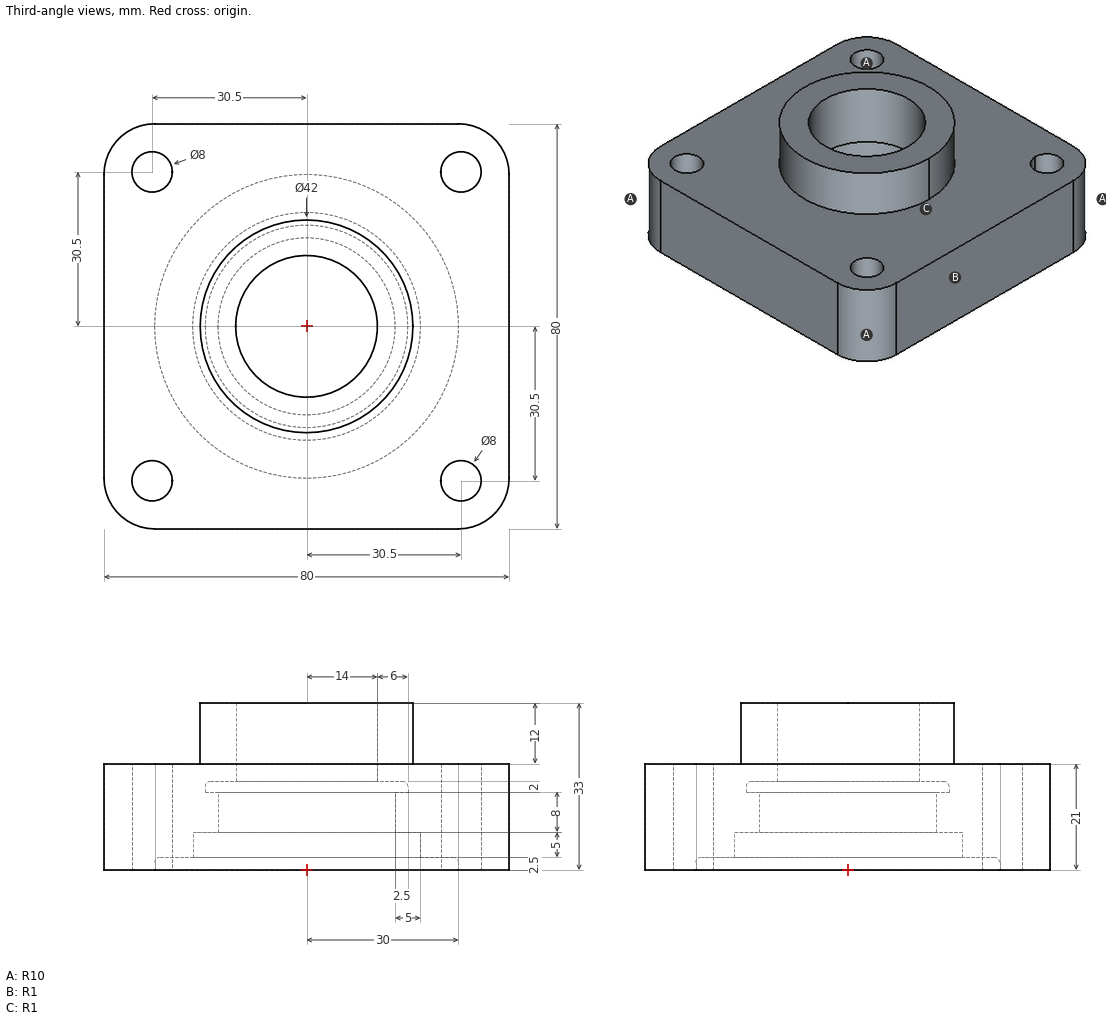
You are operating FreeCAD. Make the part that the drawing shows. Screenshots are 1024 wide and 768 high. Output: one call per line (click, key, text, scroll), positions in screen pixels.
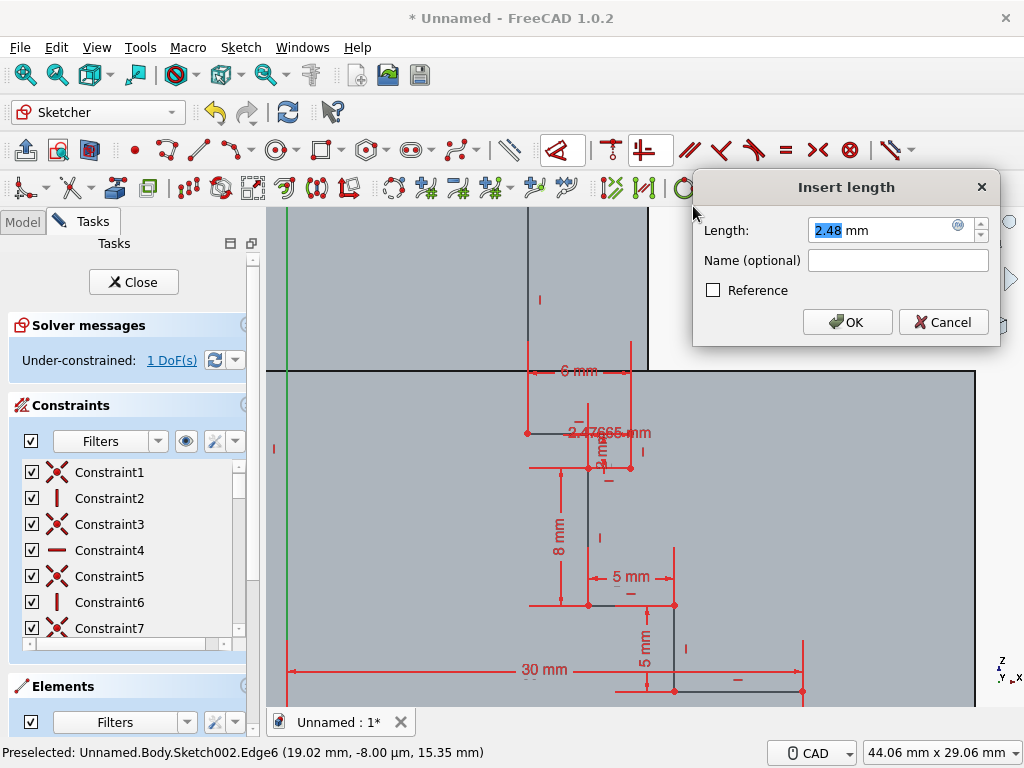
text(2.5)
key(Return)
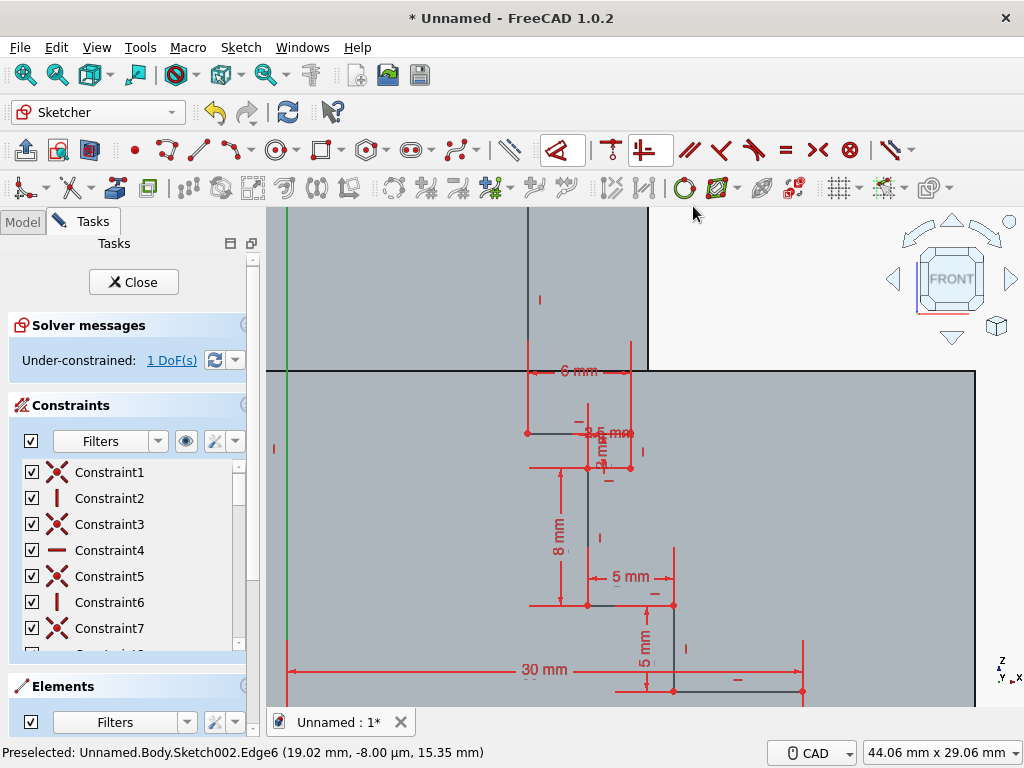
scroll(615, 467, down, 3)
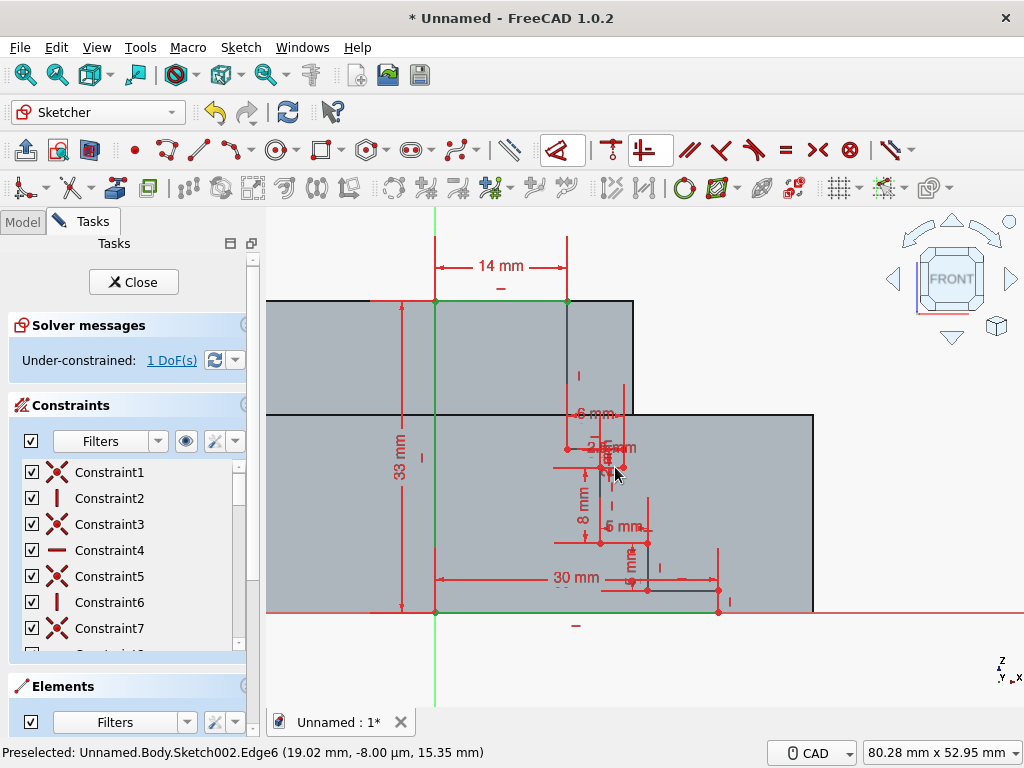
scroll(718, 597, up, 4)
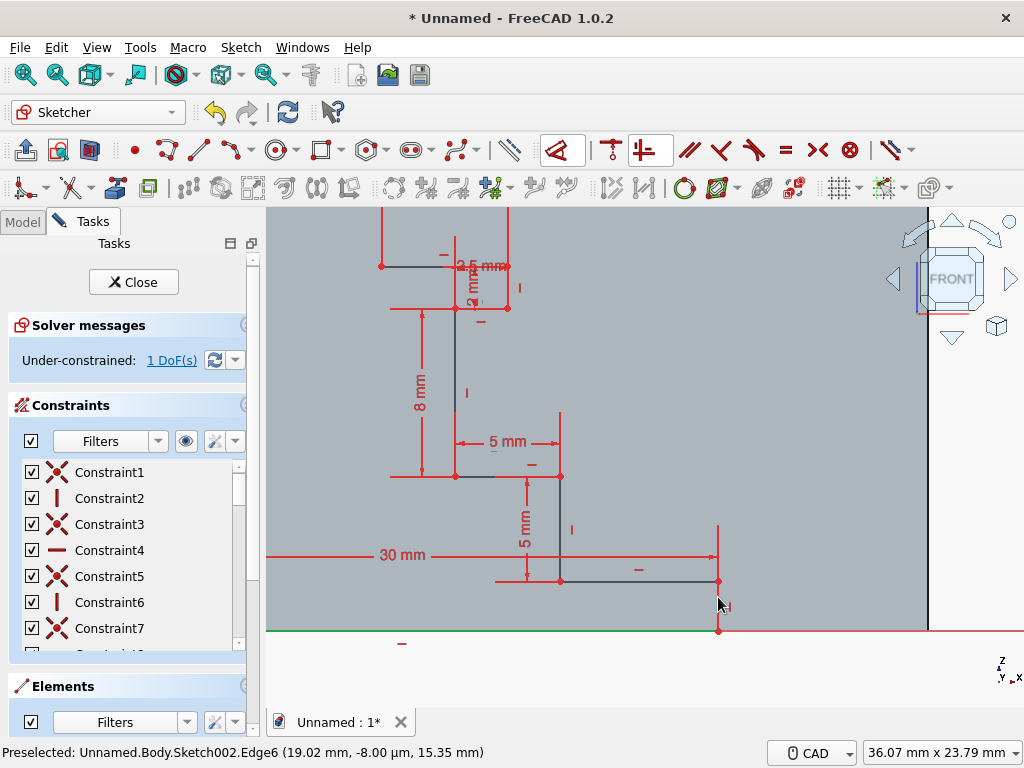
click(718, 597)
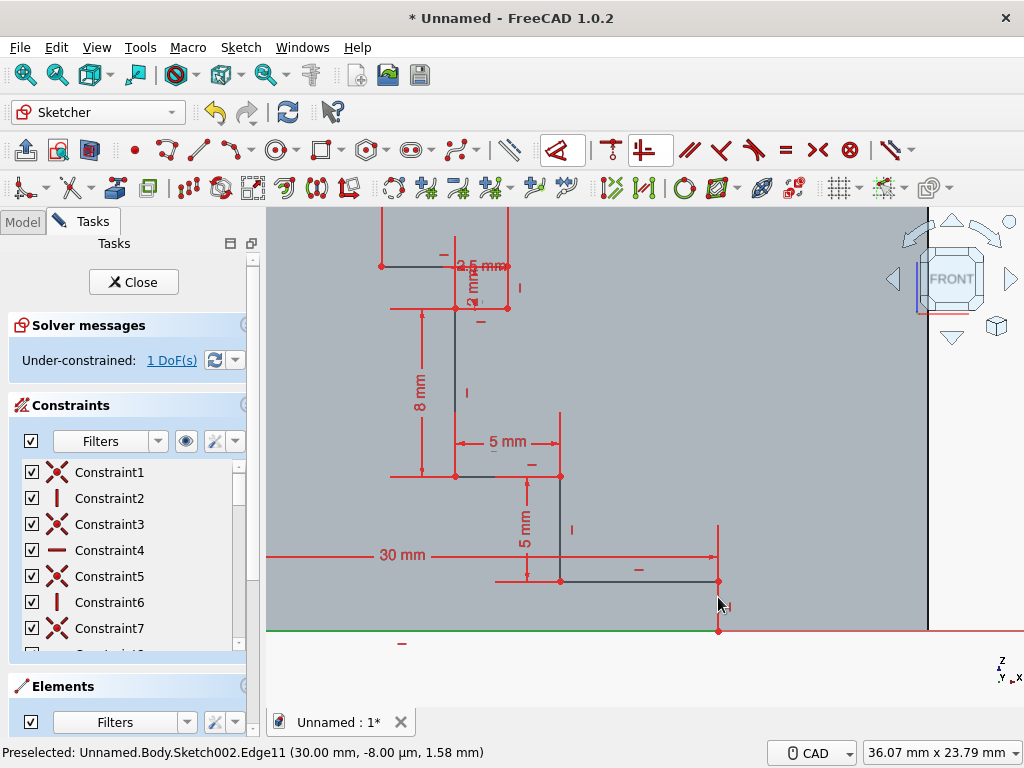
click(580, 150)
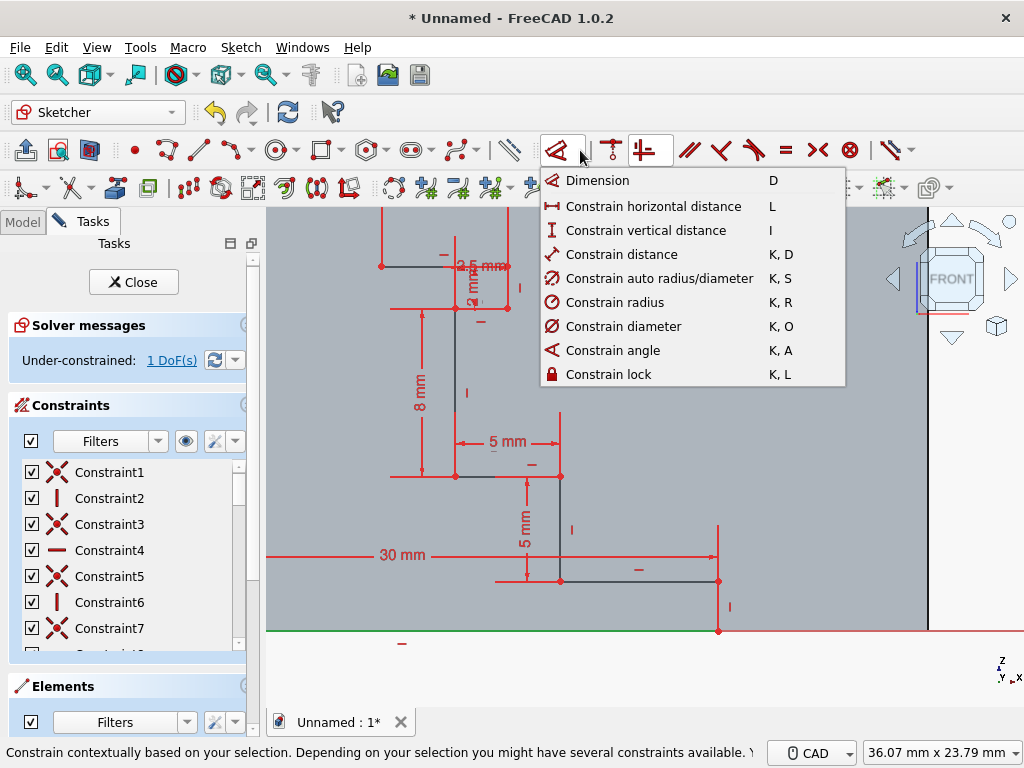
click(693, 230)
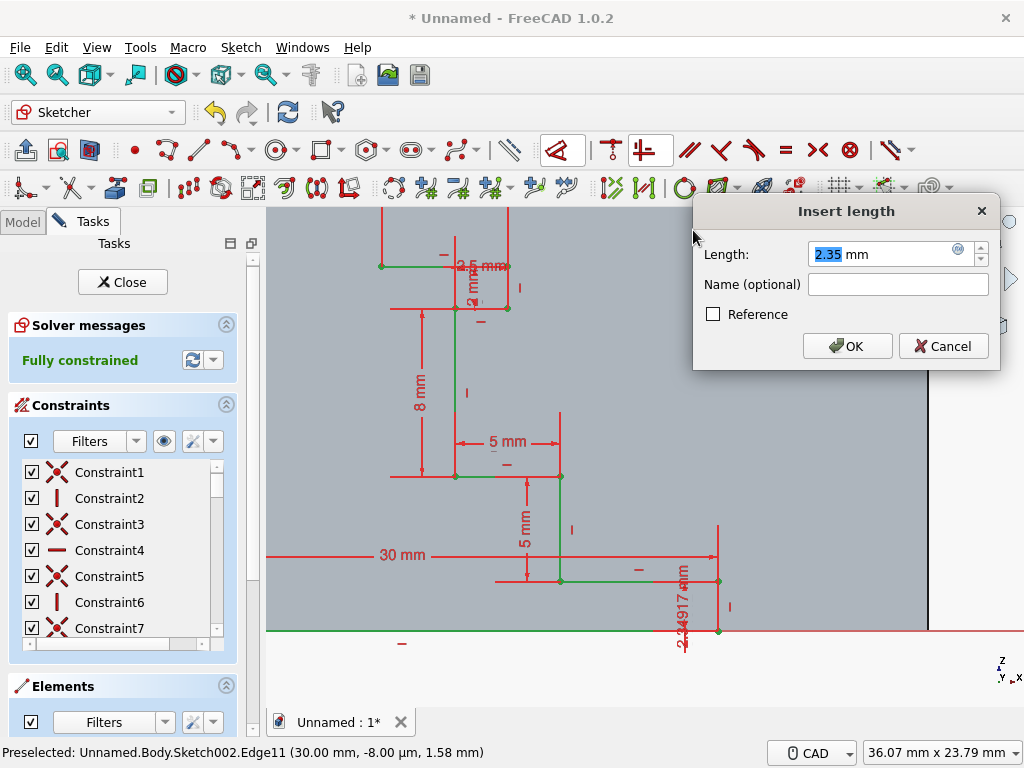
text(2.5)
key(Return)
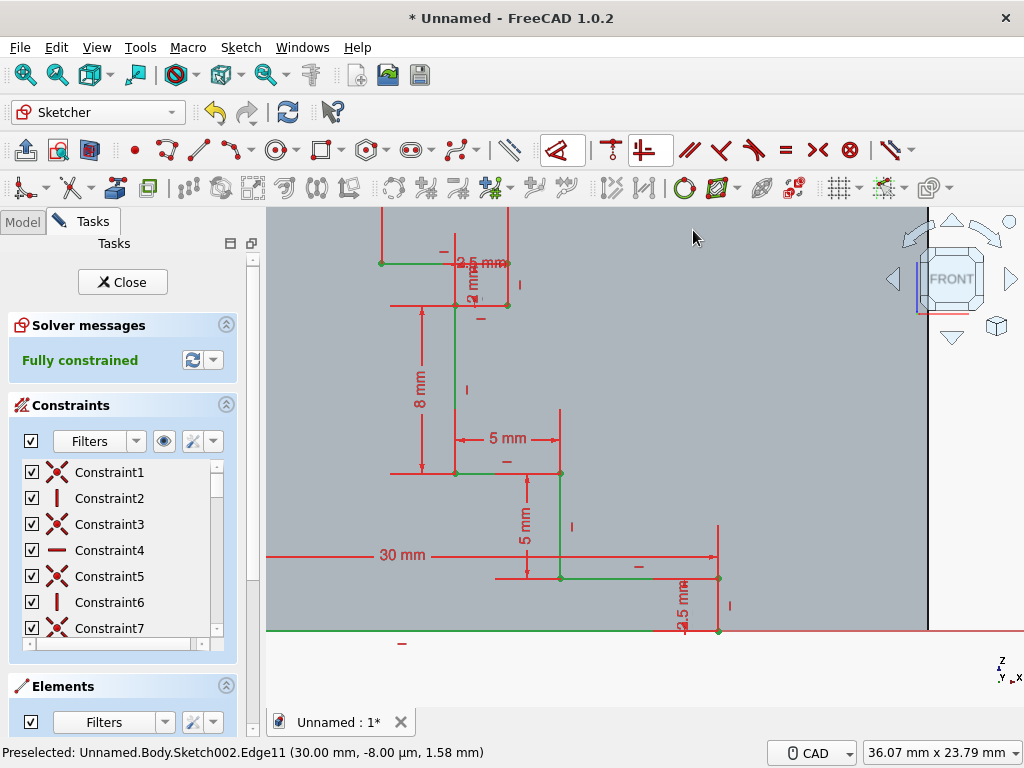
click(123, 282)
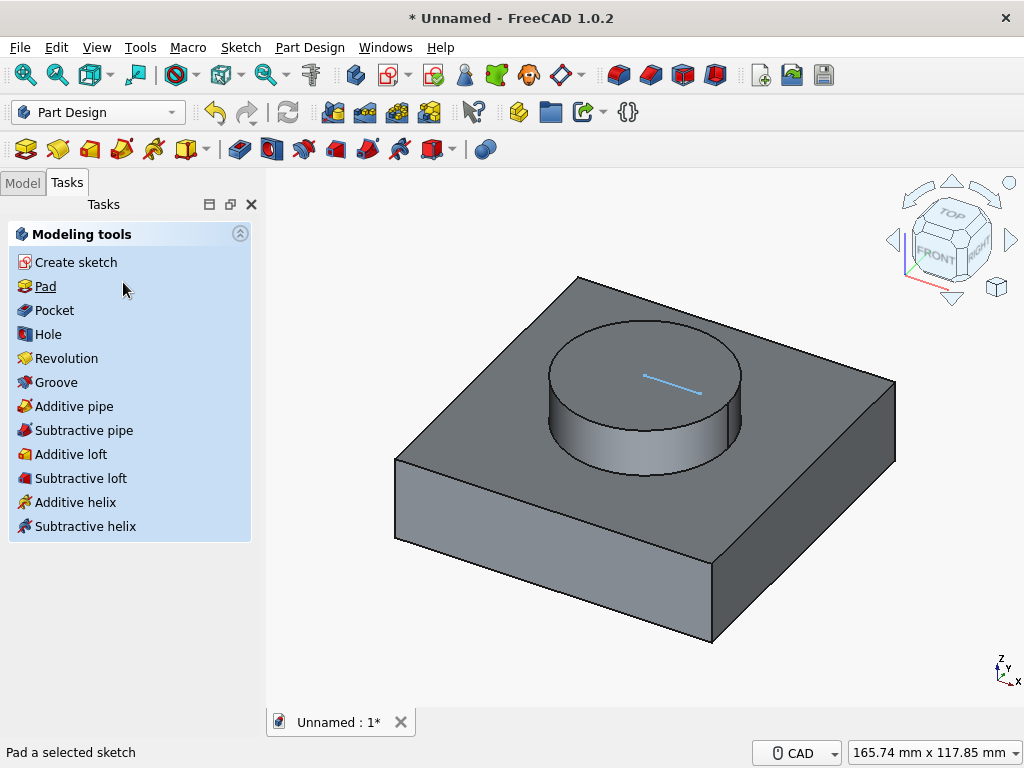
click(304, 150)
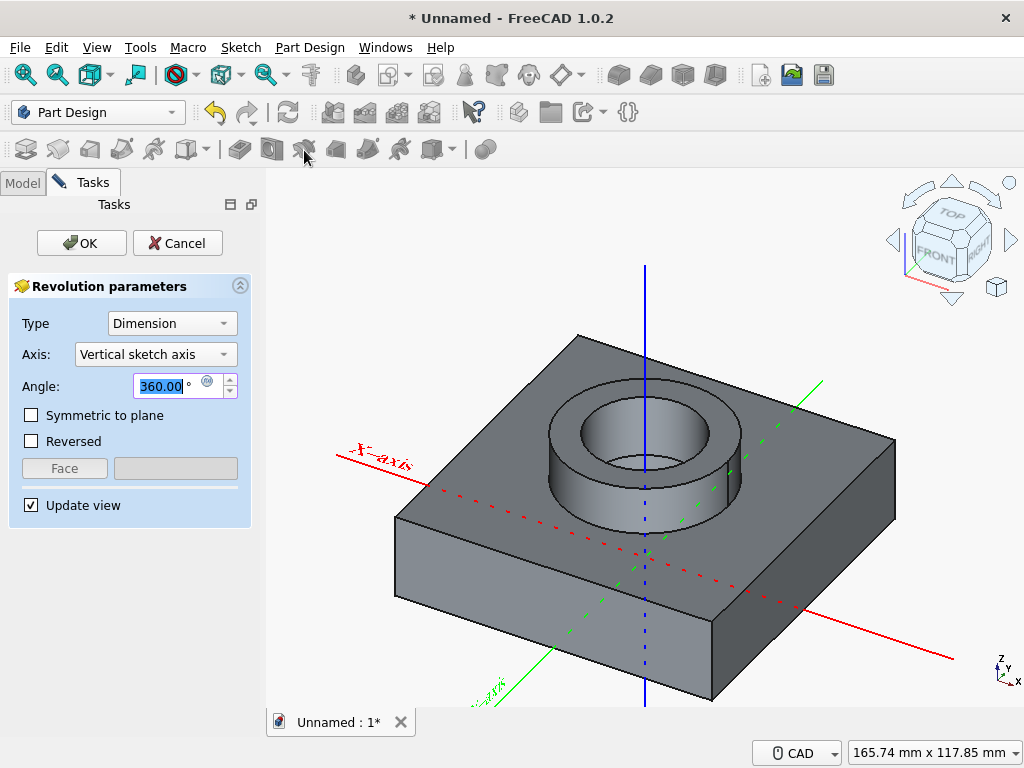
click(82, 243)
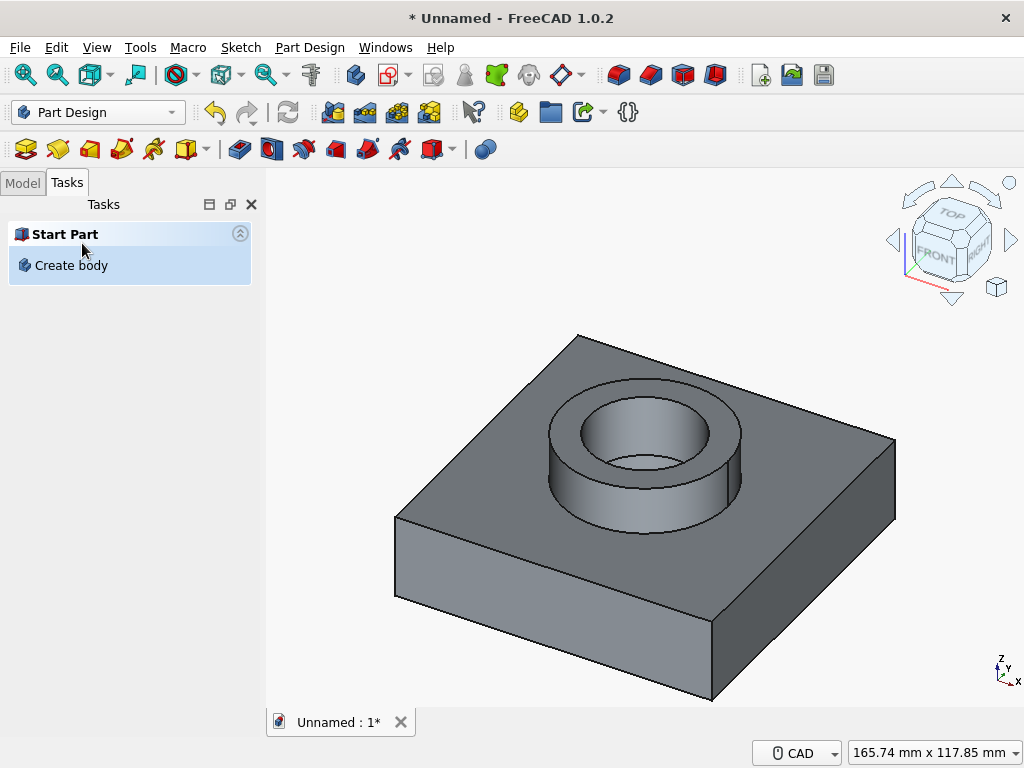
click(712, 660)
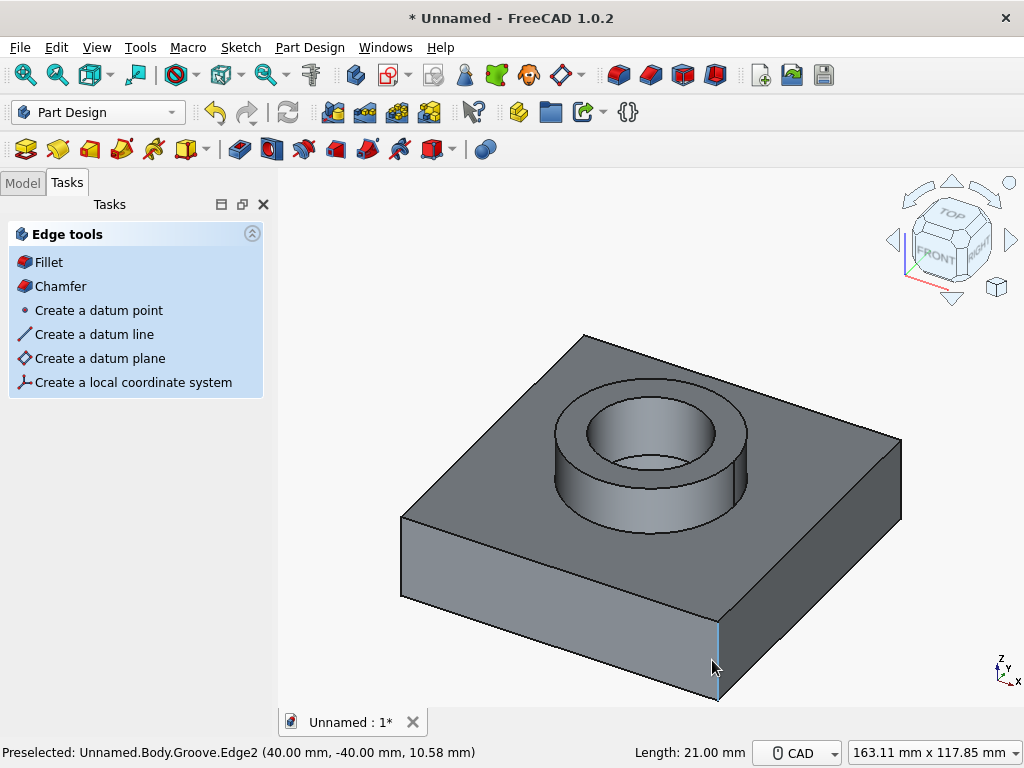
key(0)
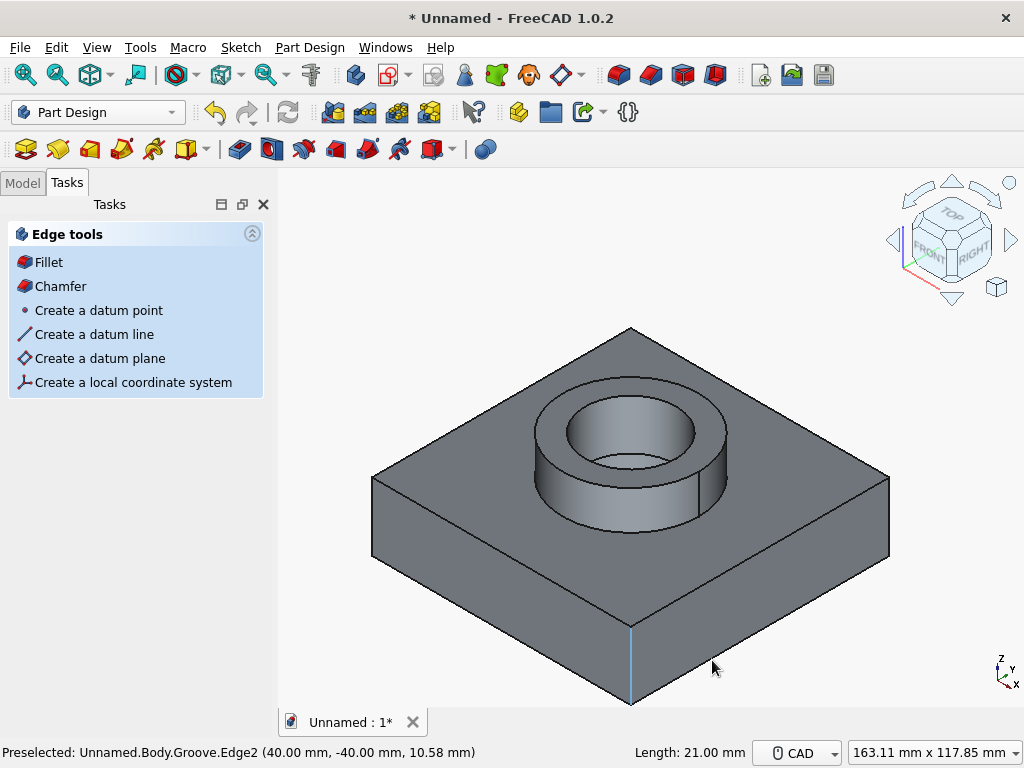
key(2)